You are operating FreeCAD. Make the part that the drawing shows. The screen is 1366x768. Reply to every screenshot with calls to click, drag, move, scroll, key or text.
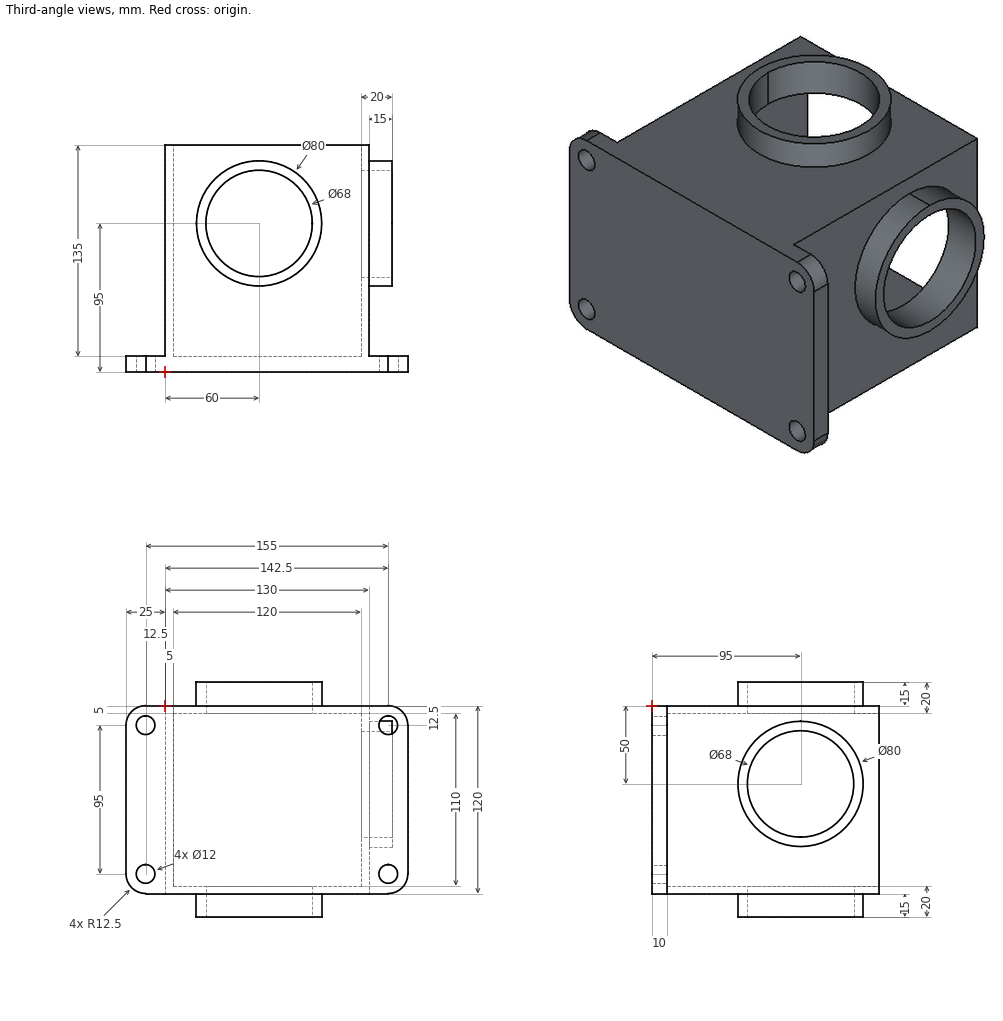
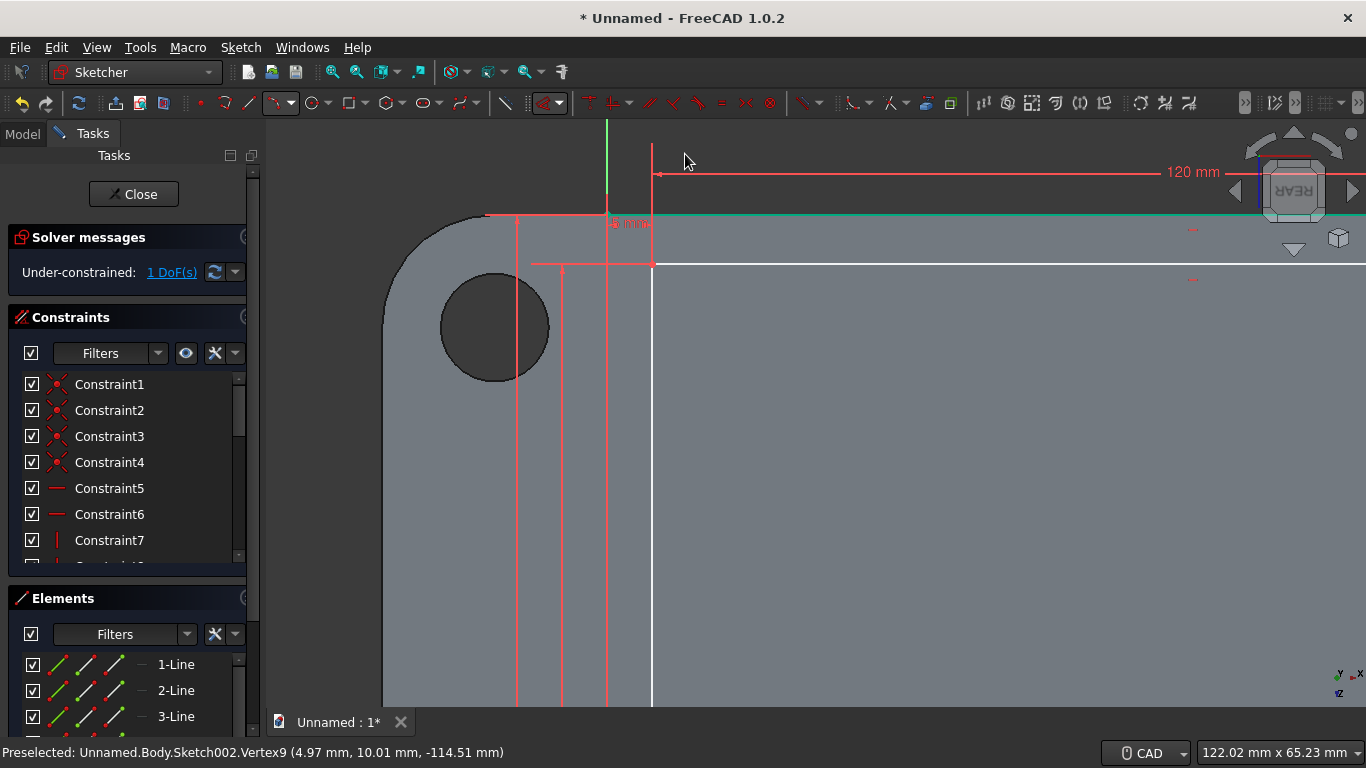
scroll(488, 213, down, 5)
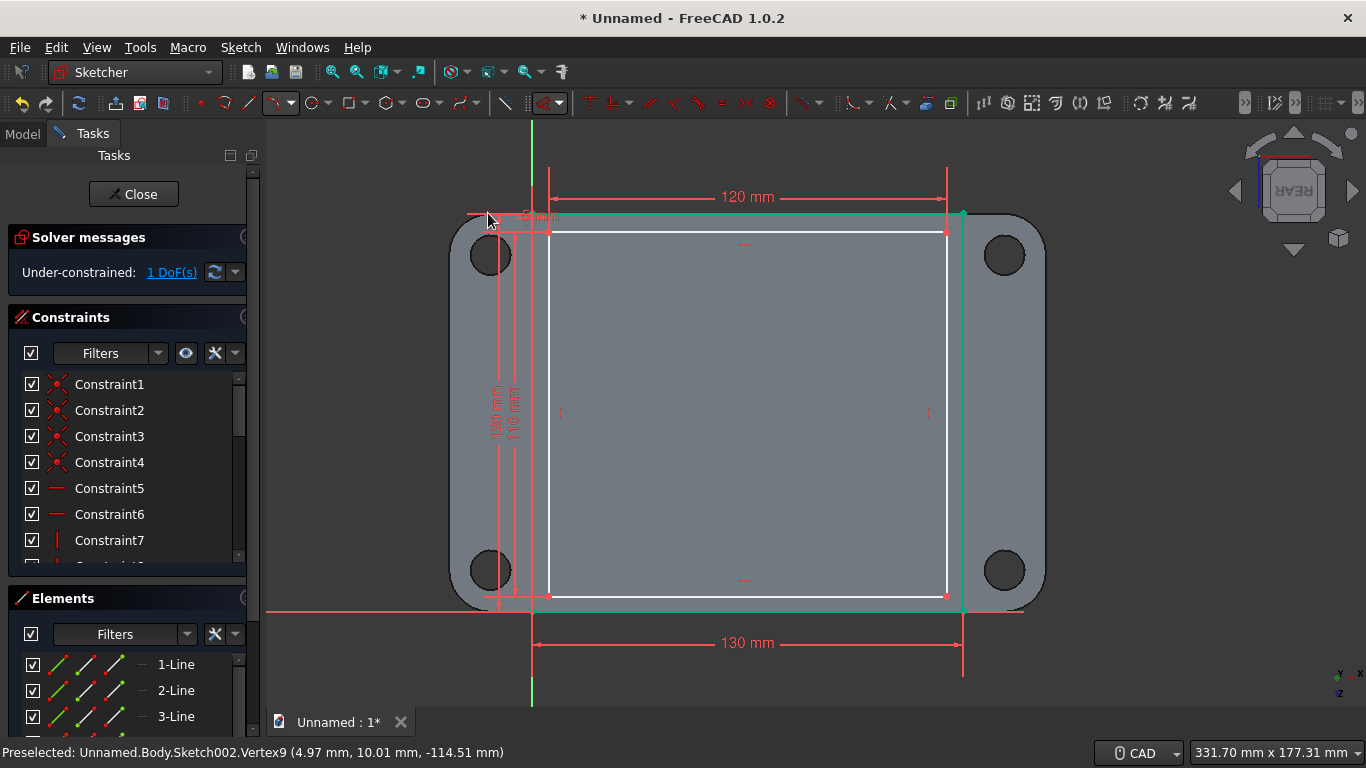
scroll(549, 597, up, 5)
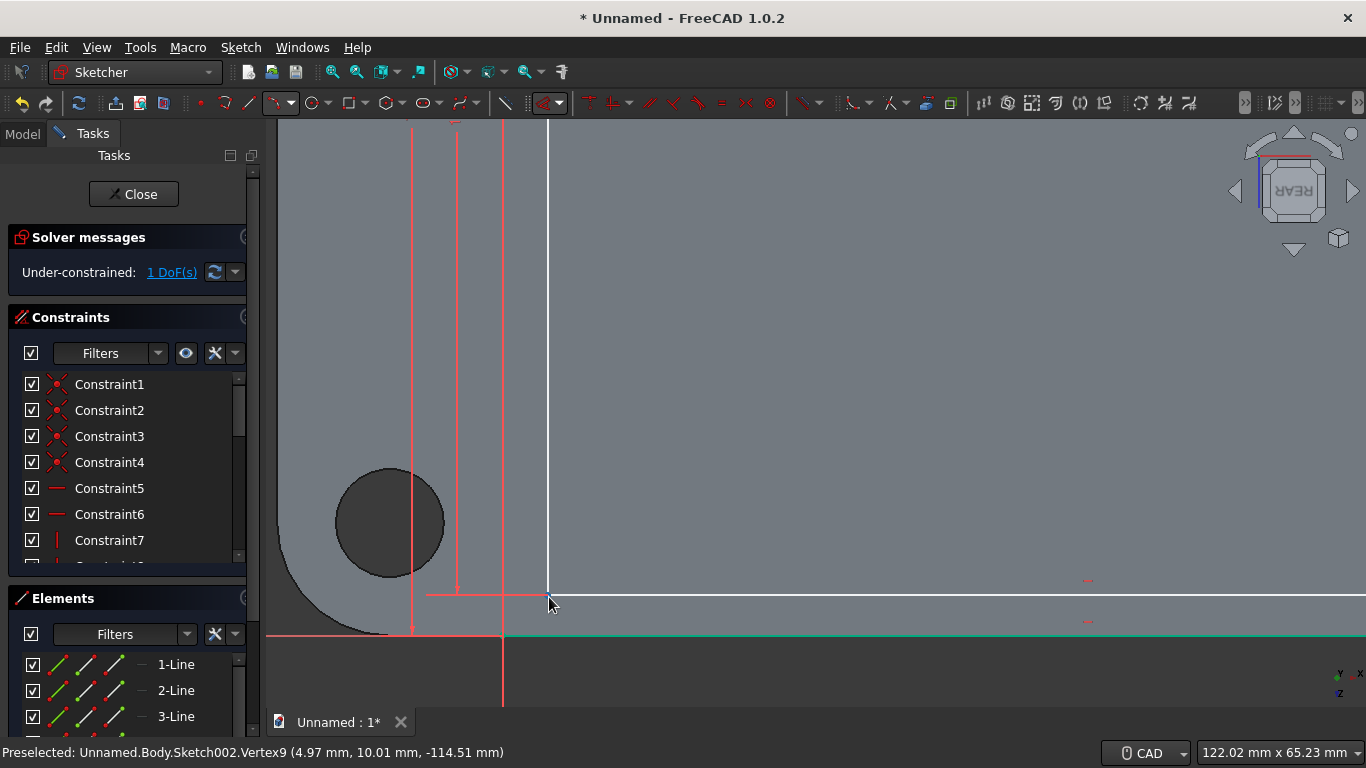
click(548, 595)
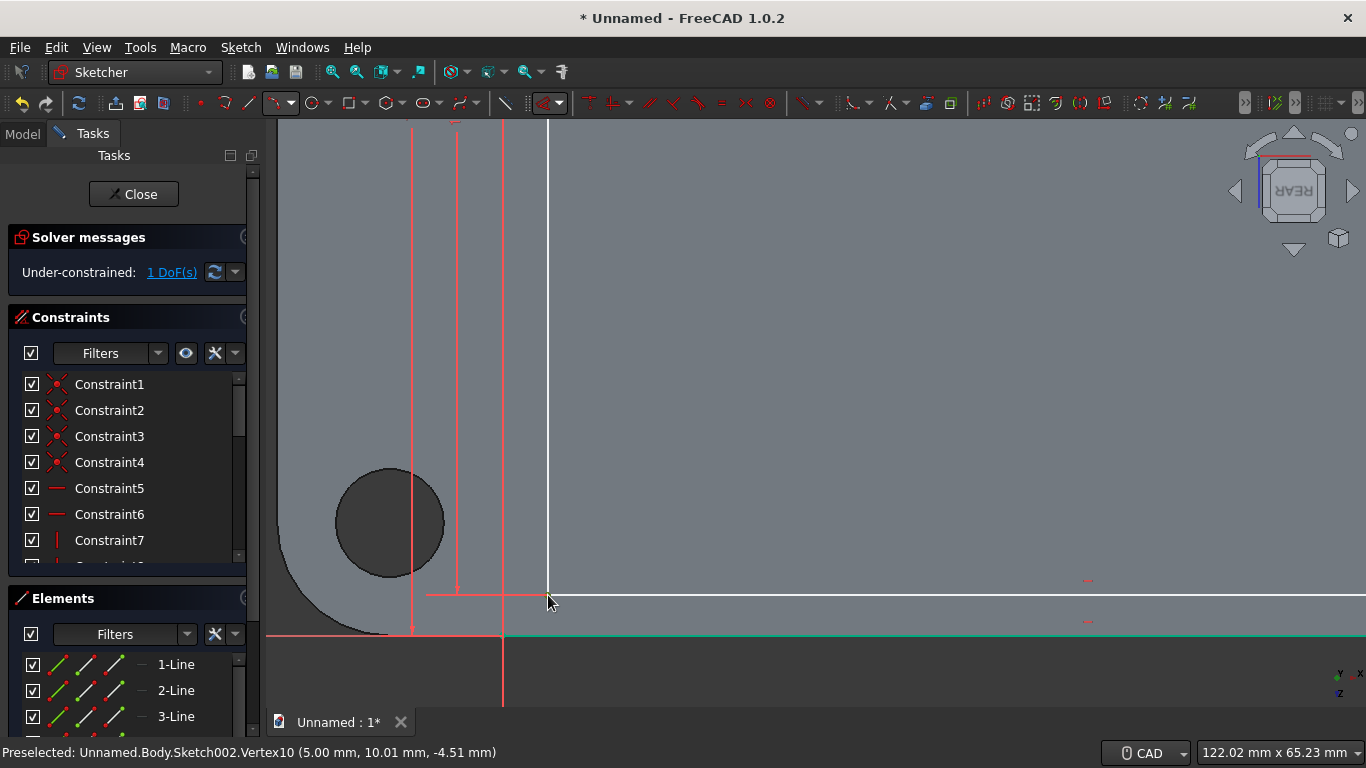
click(562, 104)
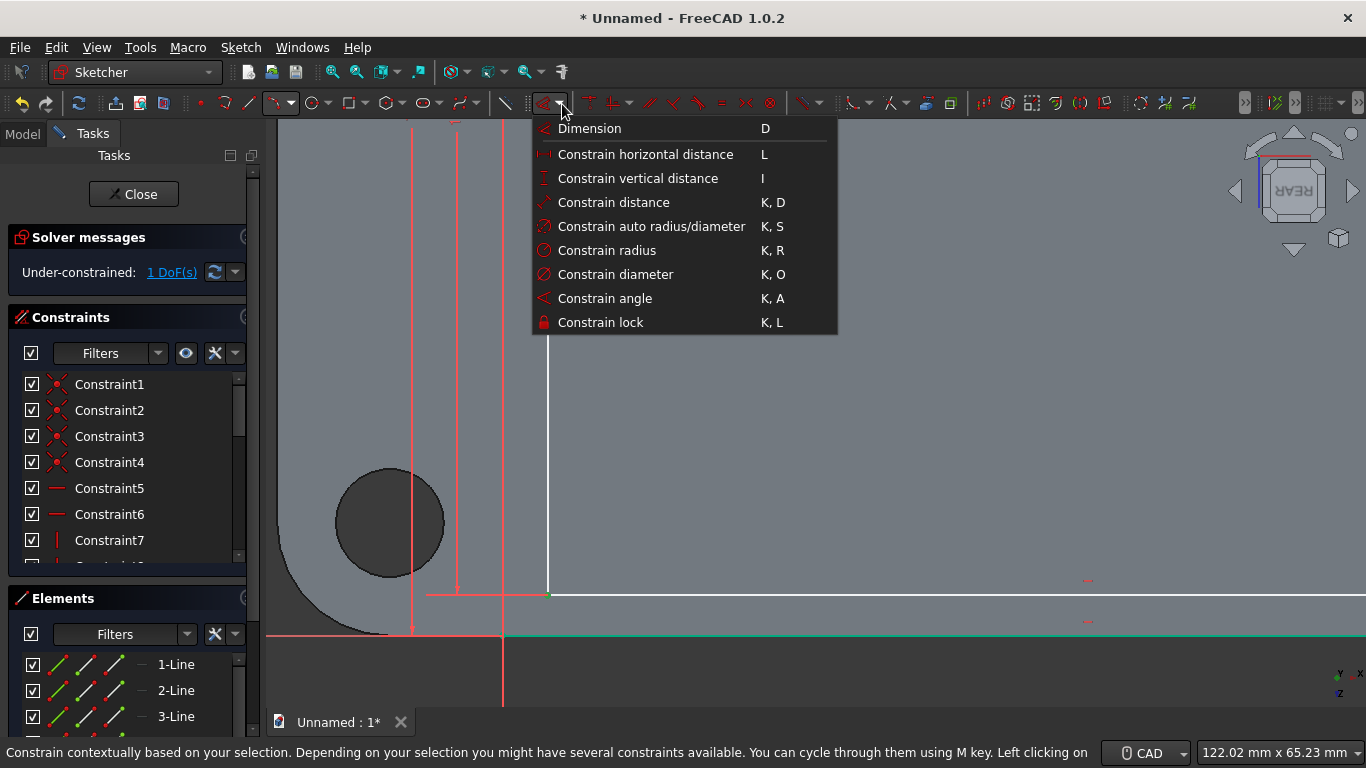
click(685, 178)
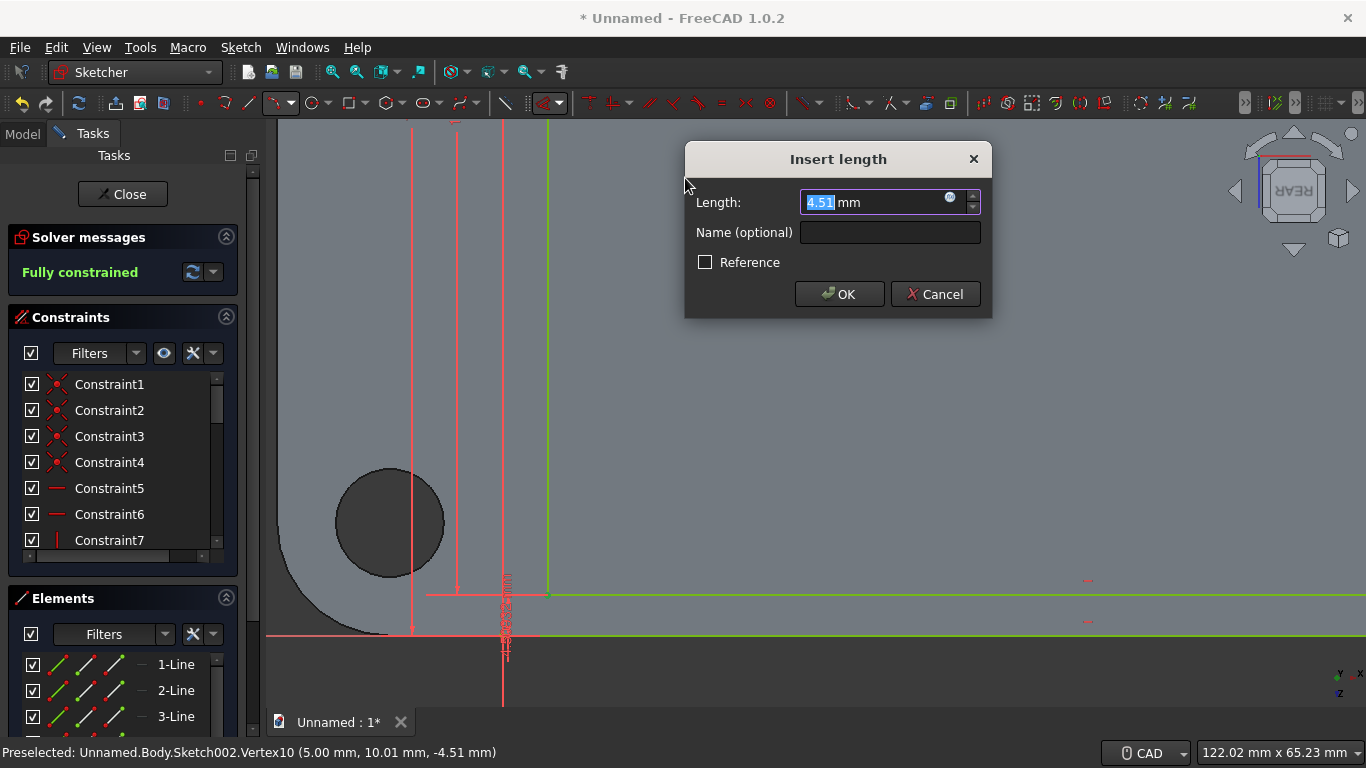
text(5)
key(Return)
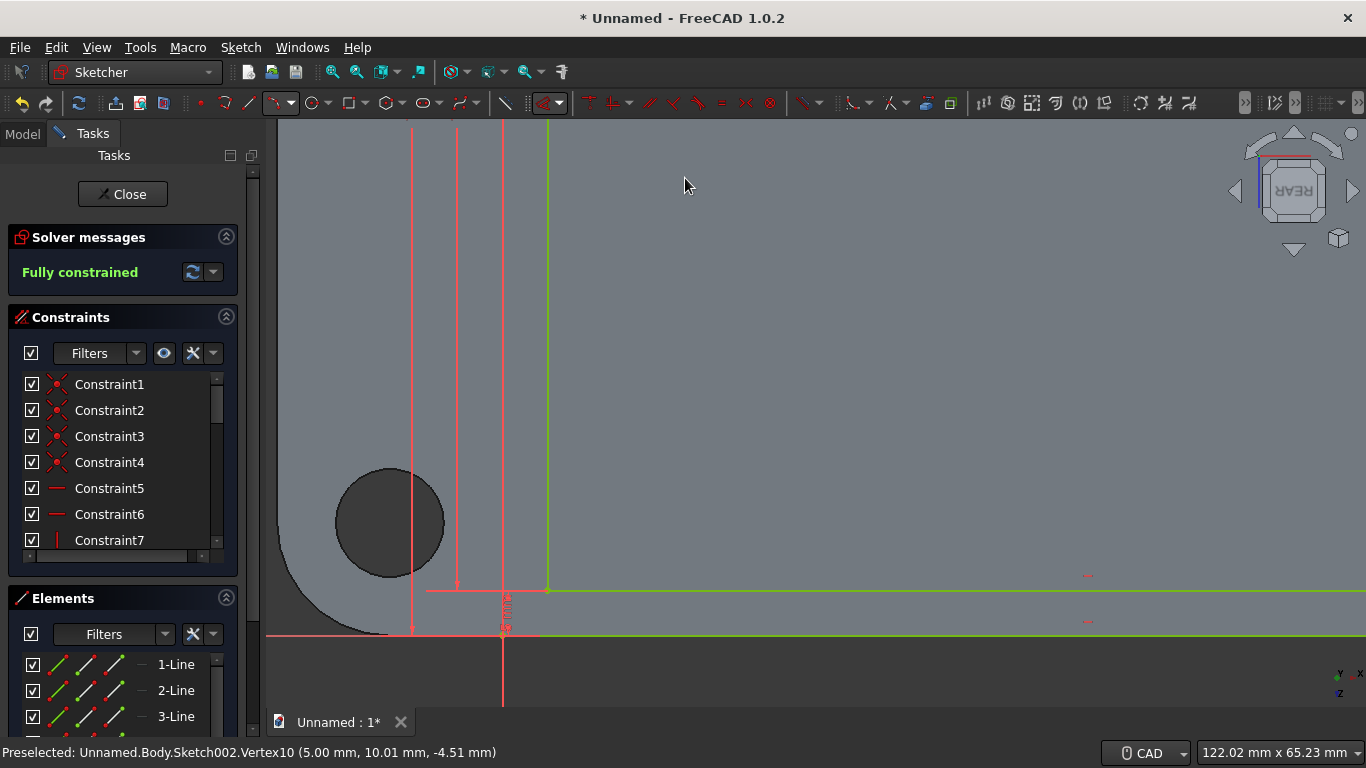
click(123, 194)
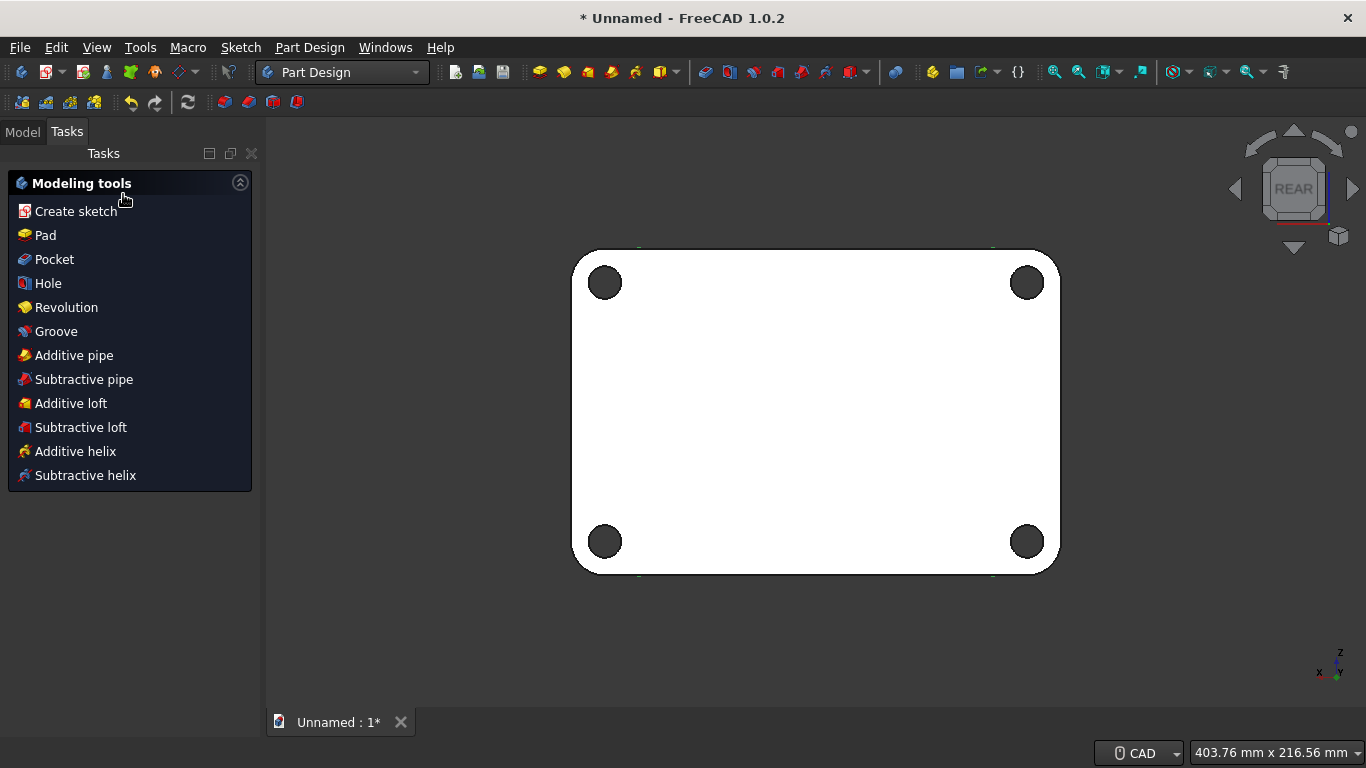
click(540, 72)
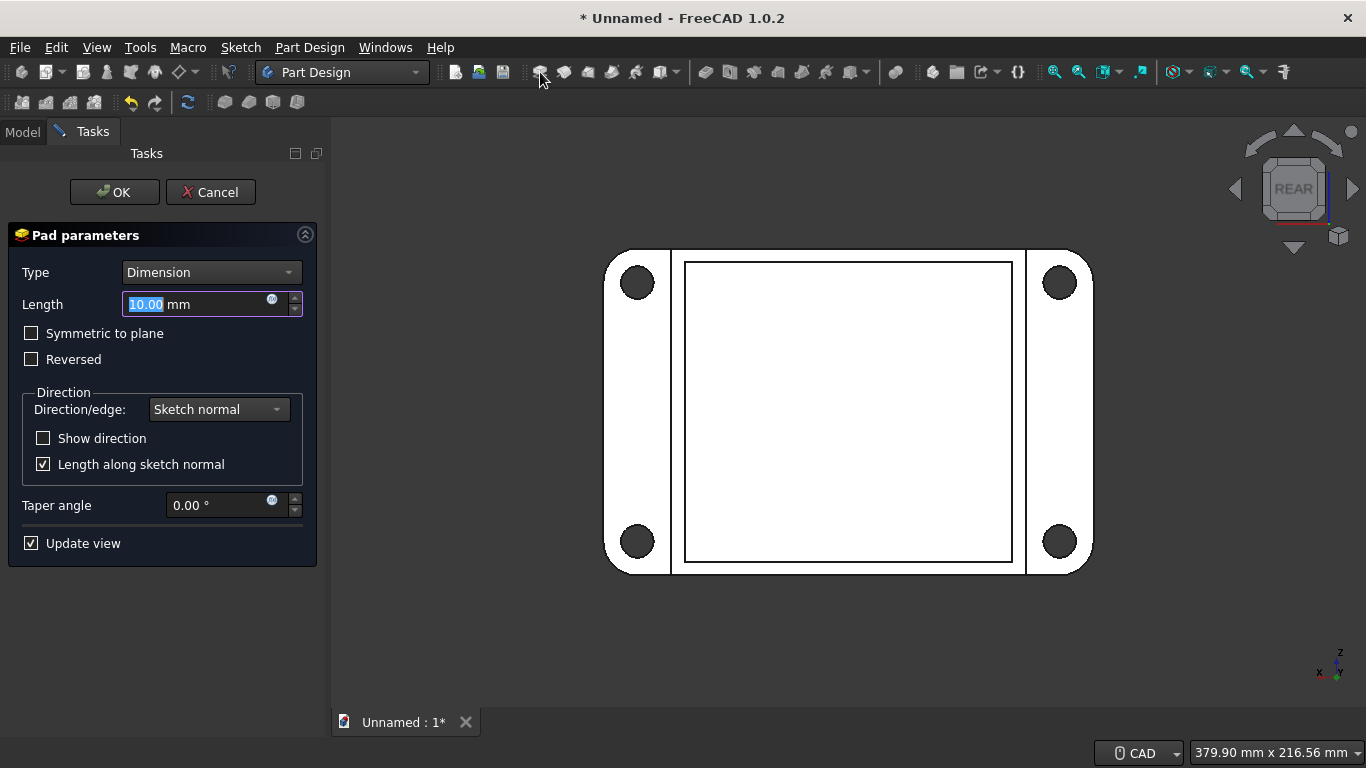
text(135)
key(Tab)